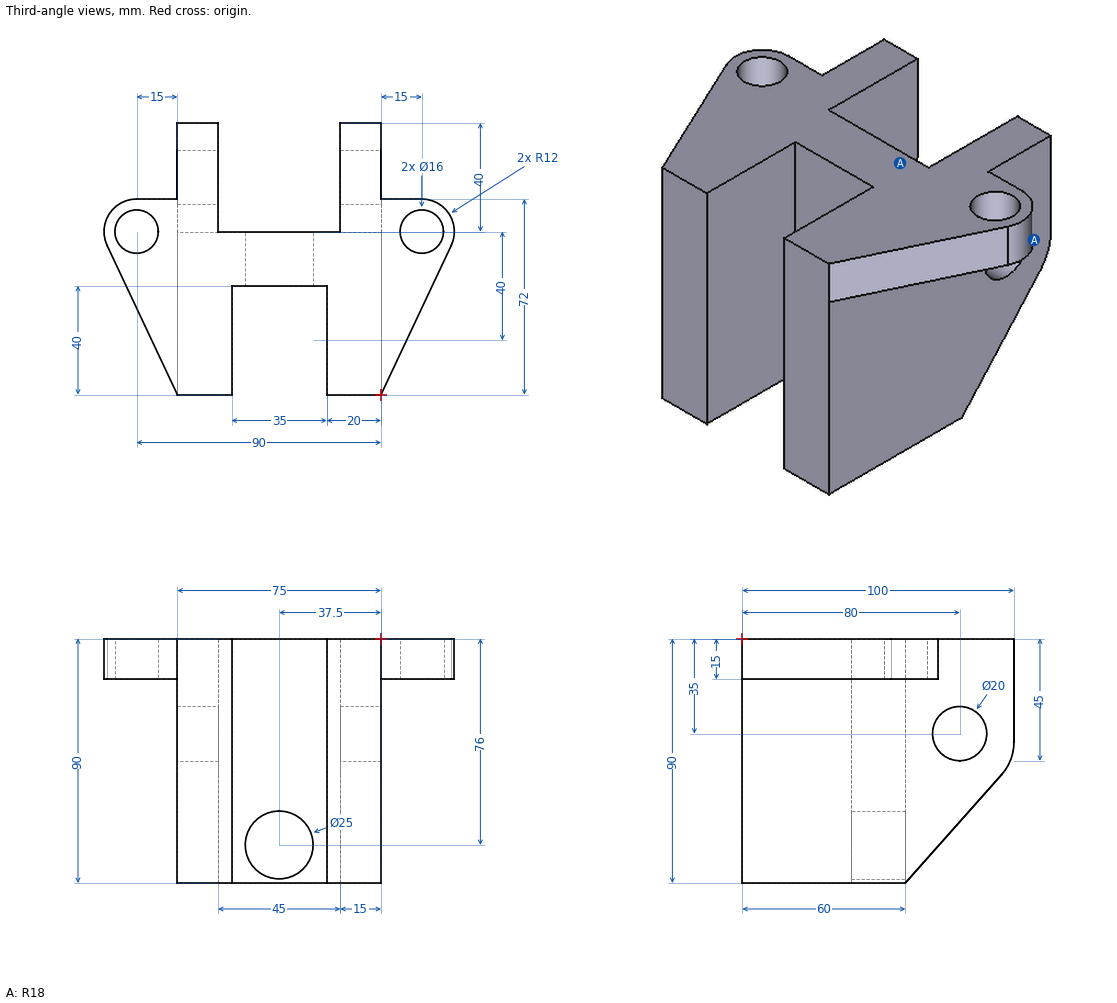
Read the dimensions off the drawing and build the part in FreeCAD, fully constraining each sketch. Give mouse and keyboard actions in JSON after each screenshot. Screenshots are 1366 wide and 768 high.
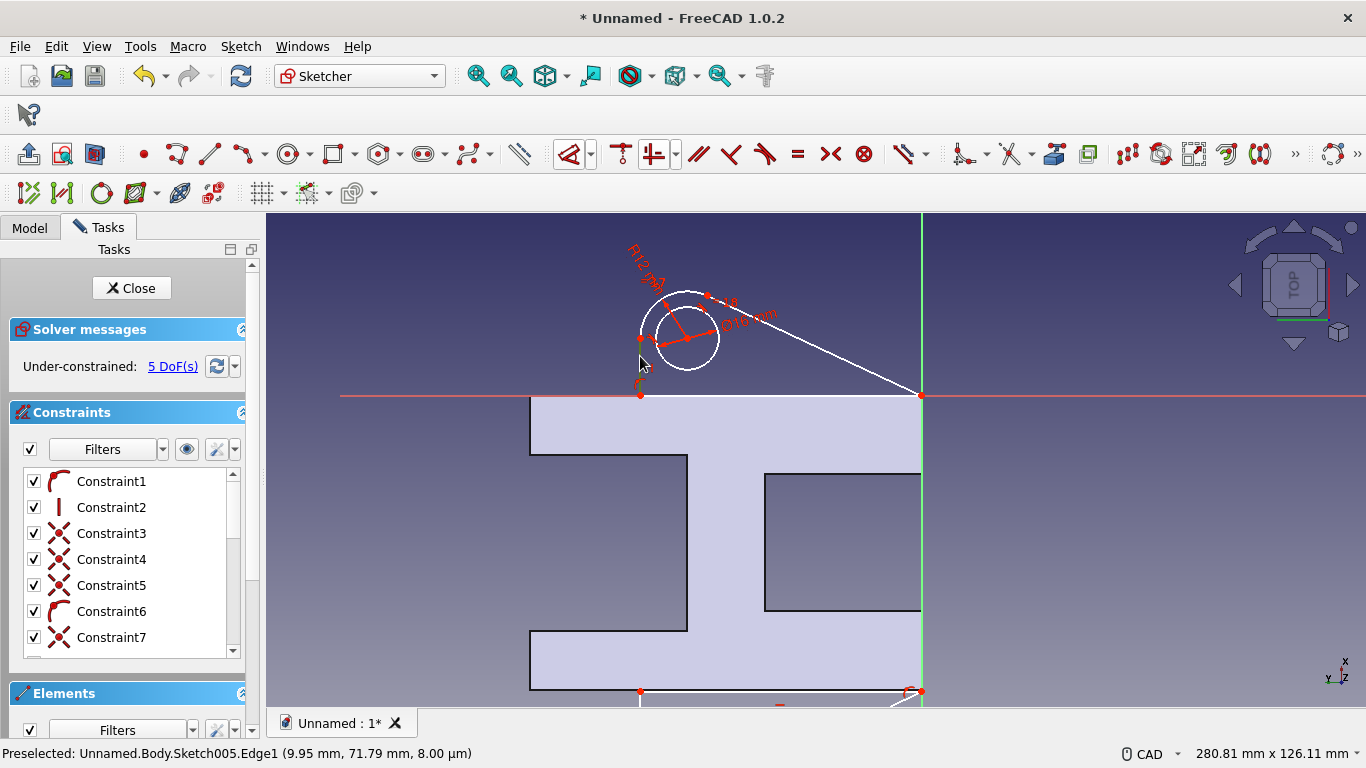
{"action": "left_click", "coordinate": [590, 154]}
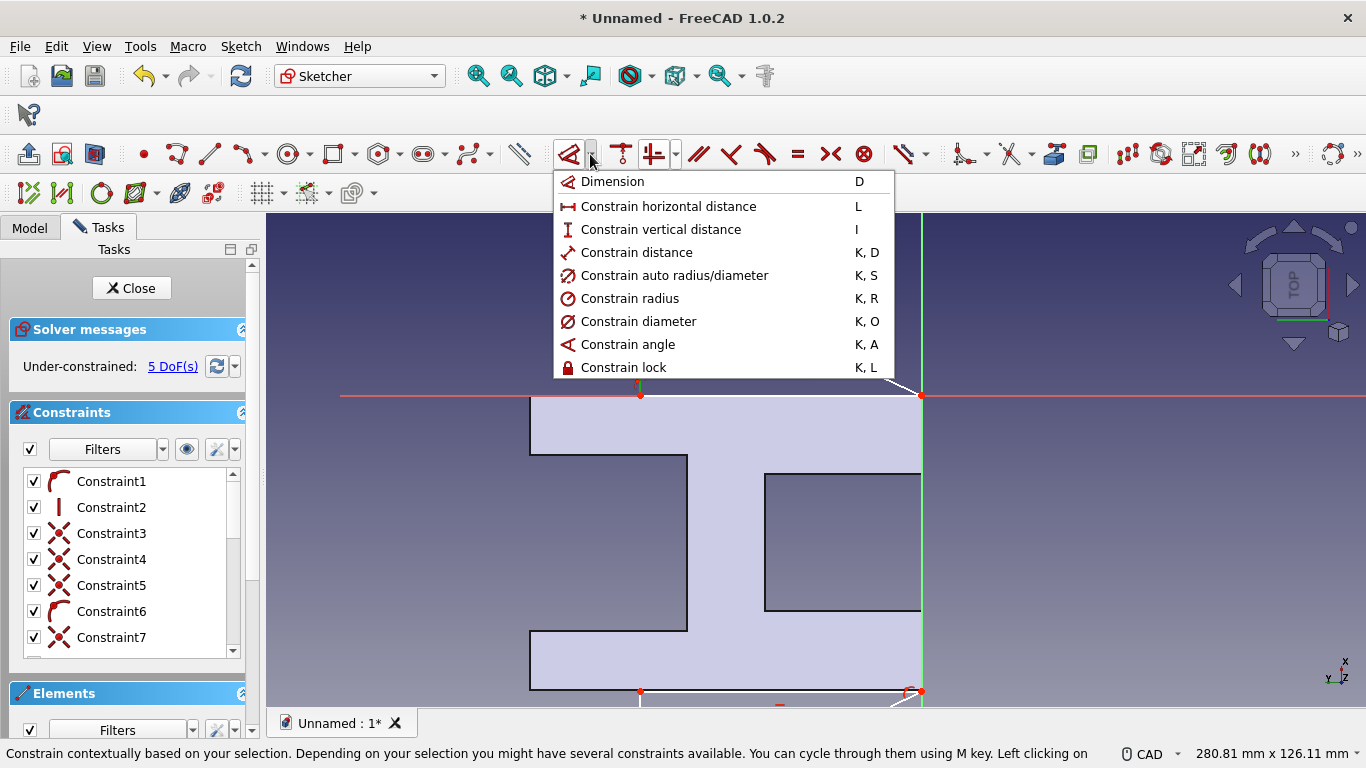
{"action": "left_click", "coordinate": [724, 230]}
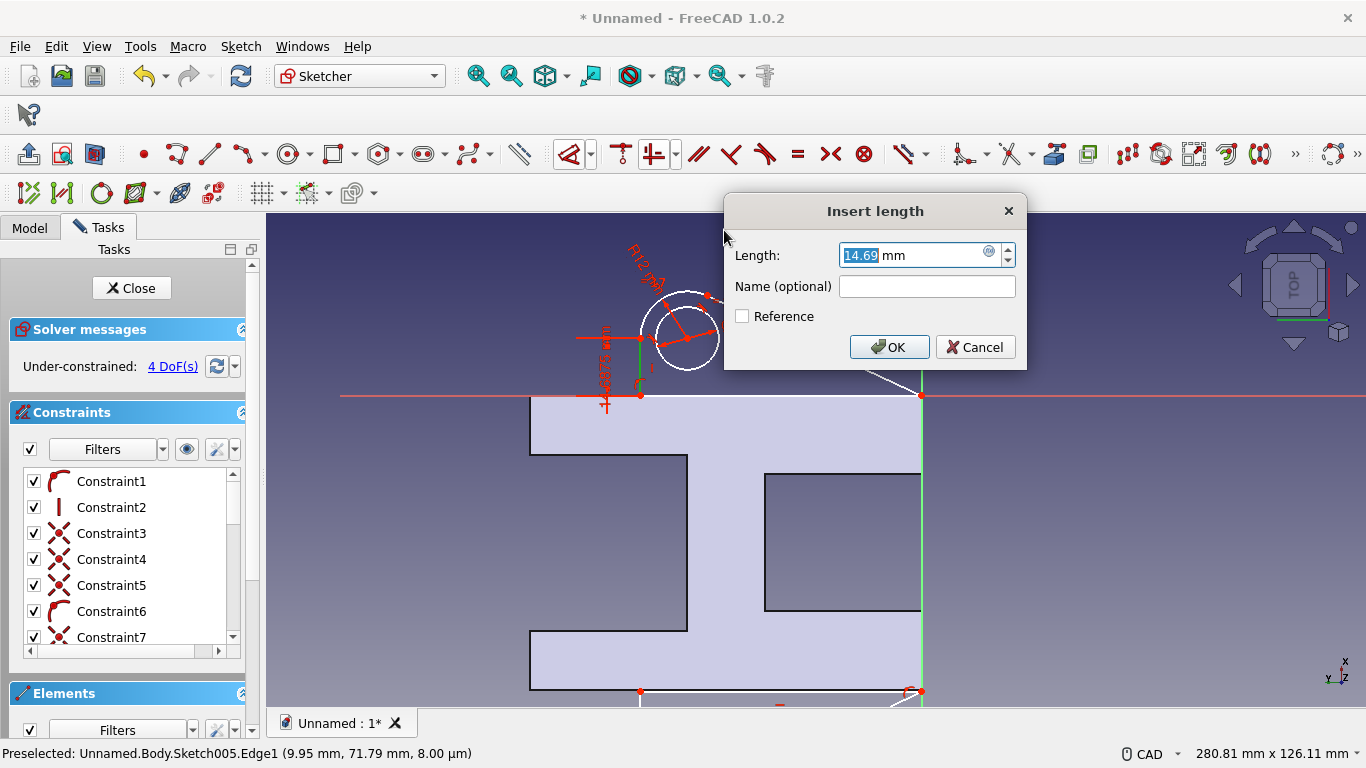
{"action": "type", "text": "15"}
{"action": "key", "text": "Return"}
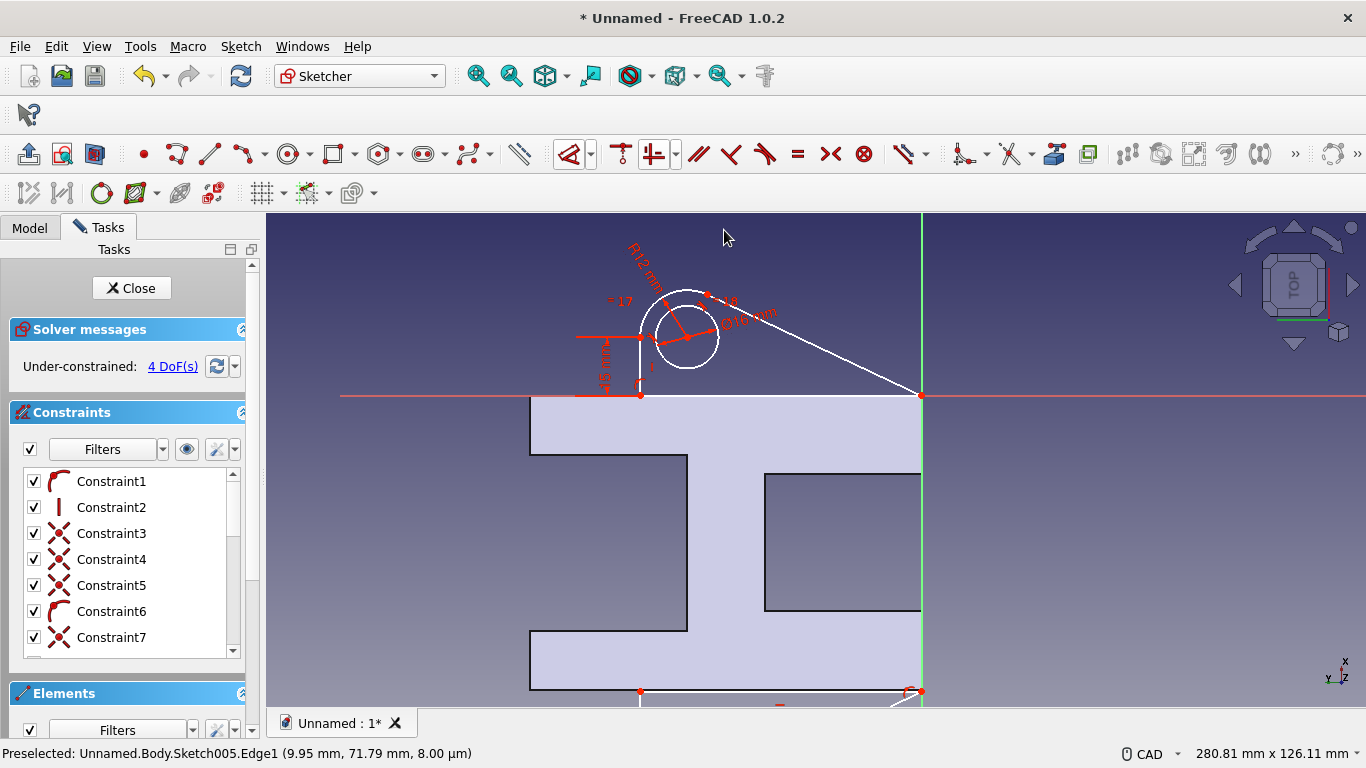
{"action": "left_click", "coordinate": [725, 396]}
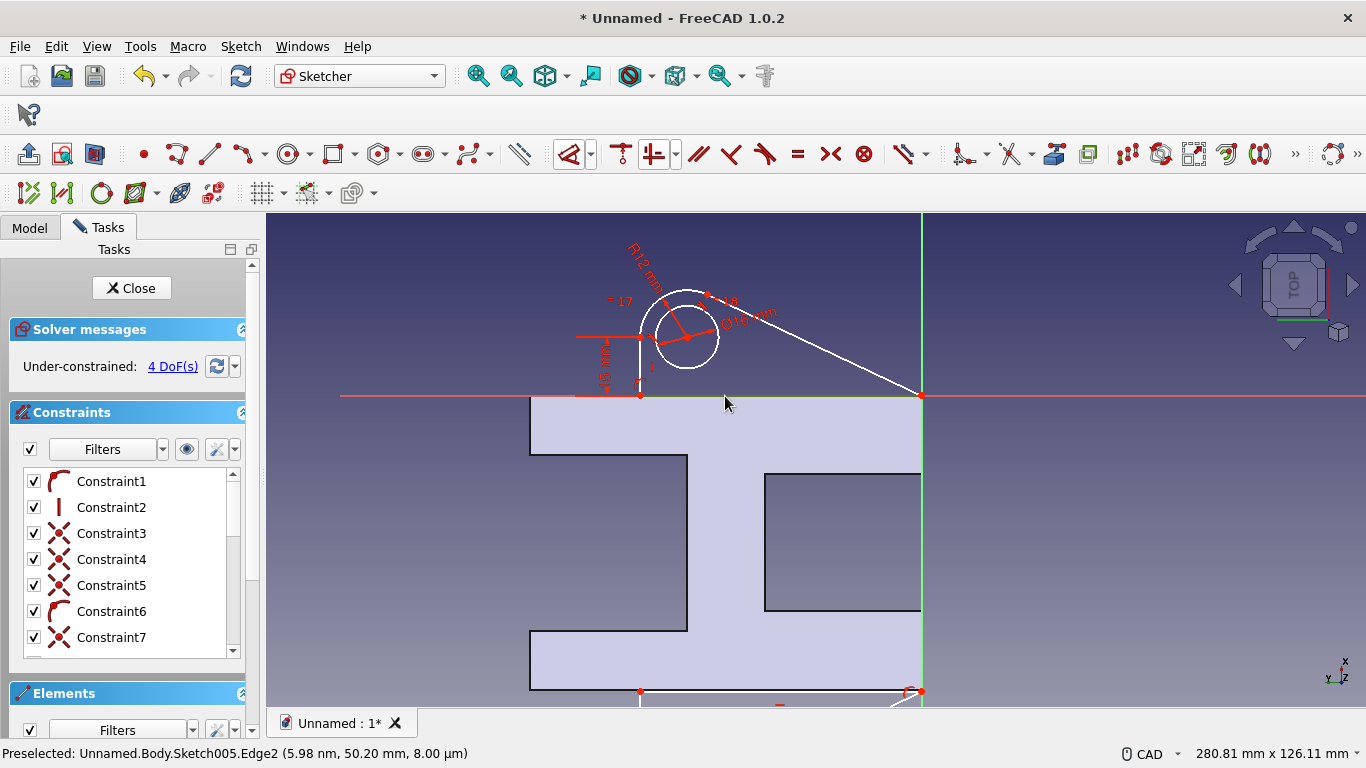
{"action": "key", "text": "l"}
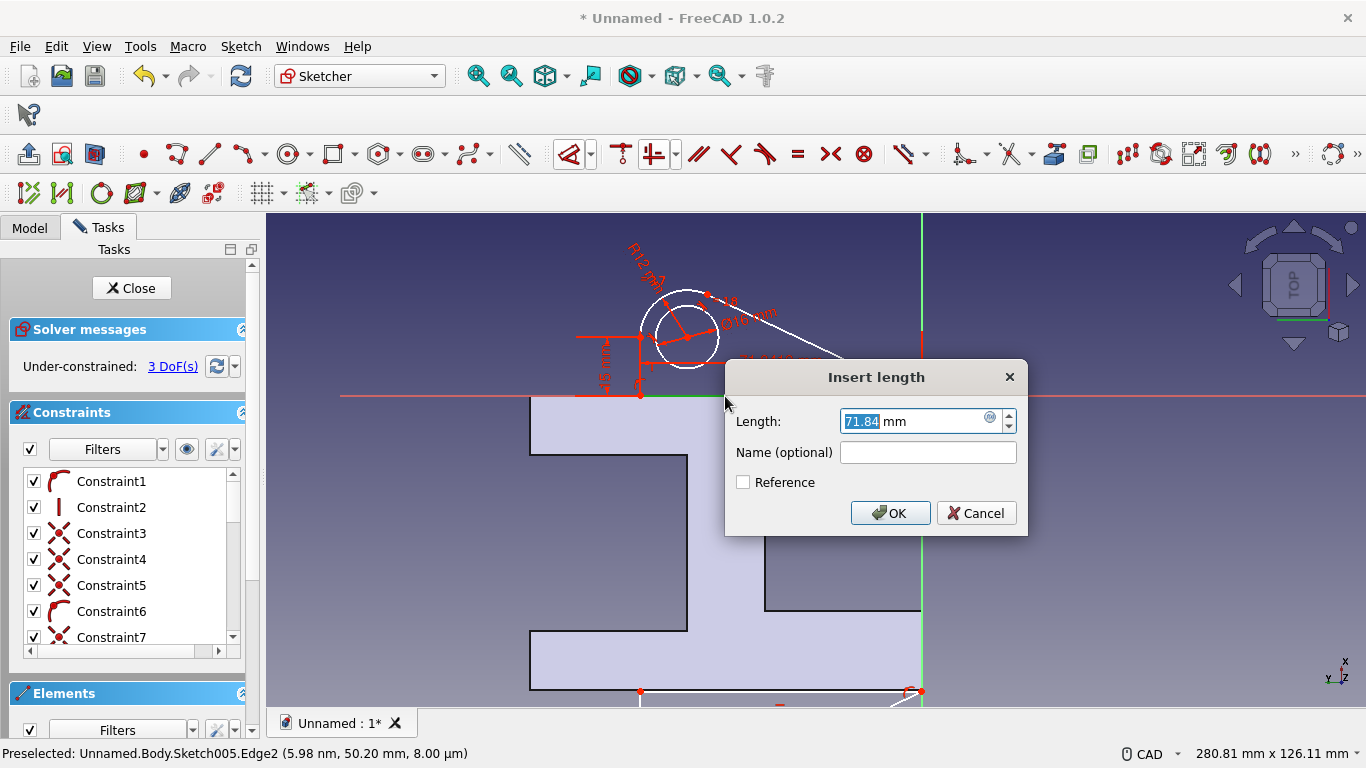
{"action": "type", "text": "72"}
{"action": "key", "text": "Return"}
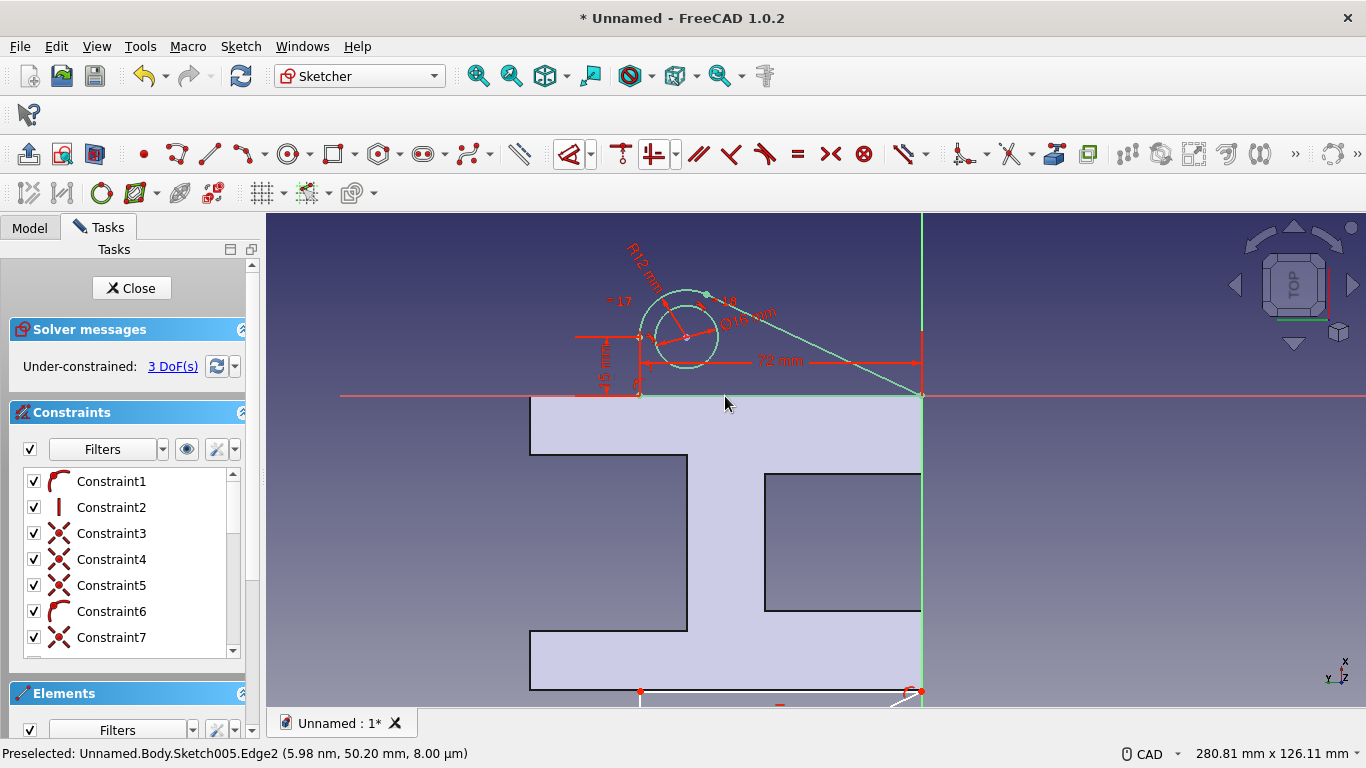
{"action": "scroll", "coordinate": [680, 292], "scroll_direction": "down", "scroll_amount": 2}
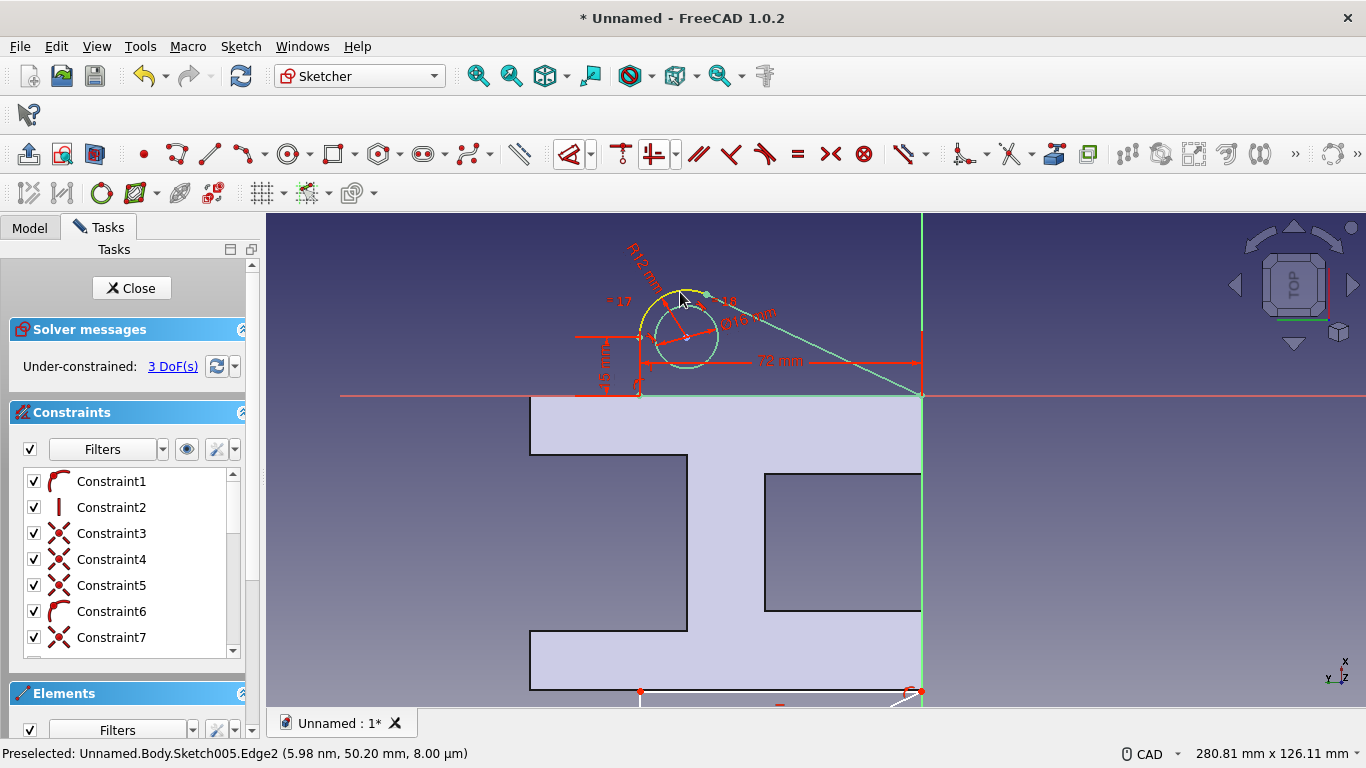
{"action": "left_click", "coordinate": [786, 560]}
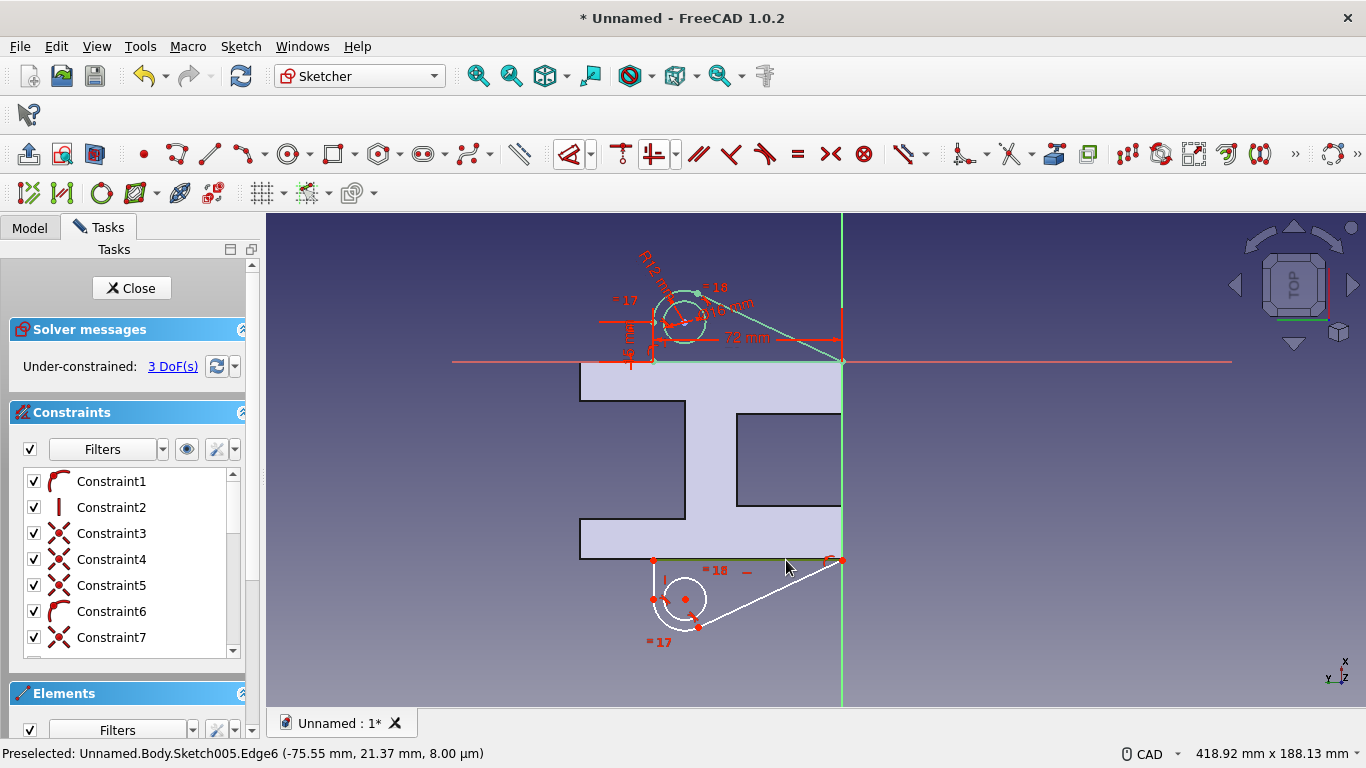
{"action": "key", "text": "l"}